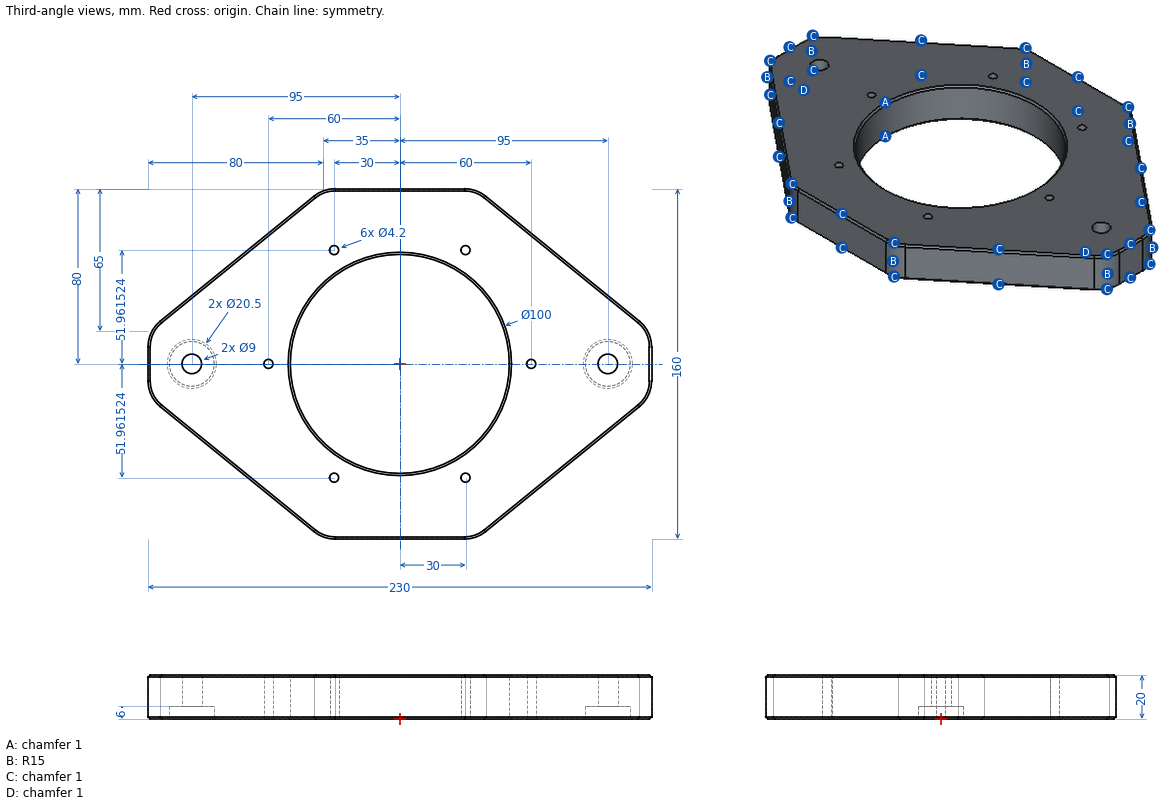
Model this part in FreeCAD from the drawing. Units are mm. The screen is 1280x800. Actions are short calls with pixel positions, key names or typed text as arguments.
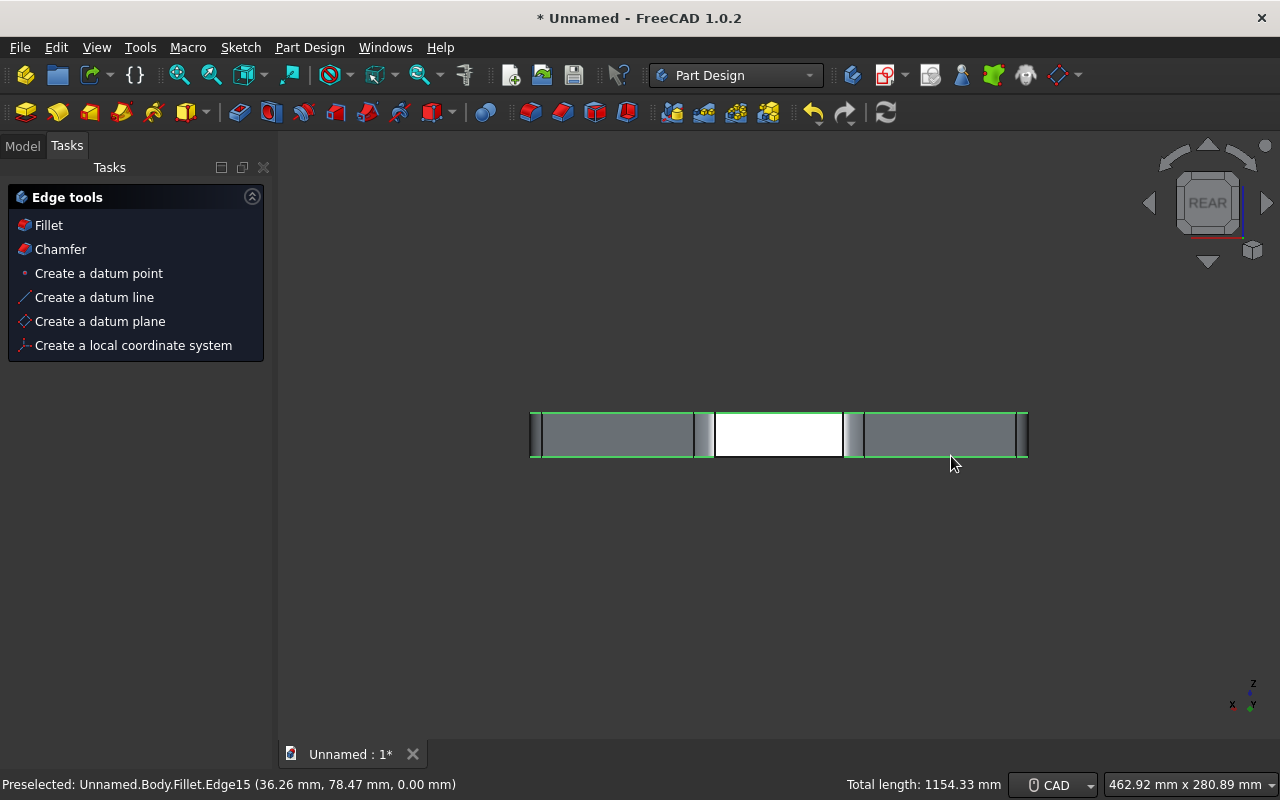
click(779, 456, ctrl)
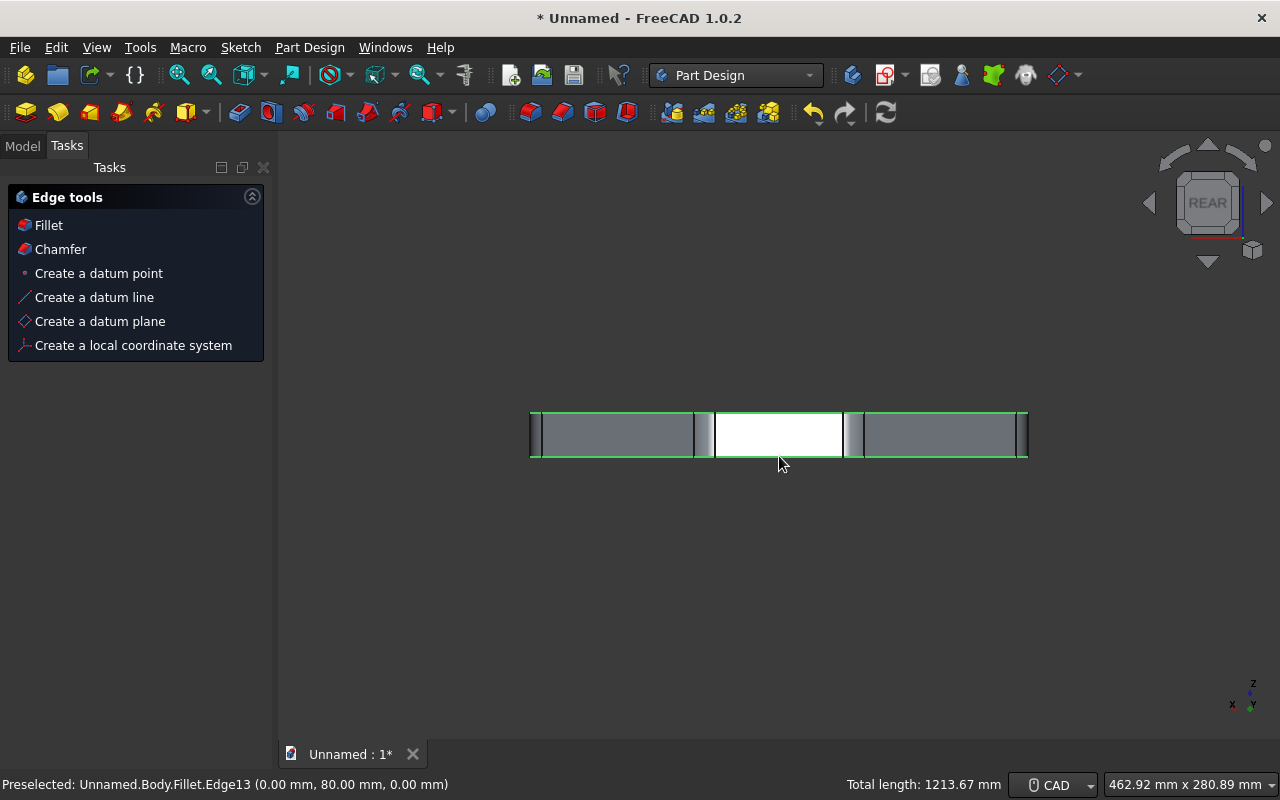
click(564, 112)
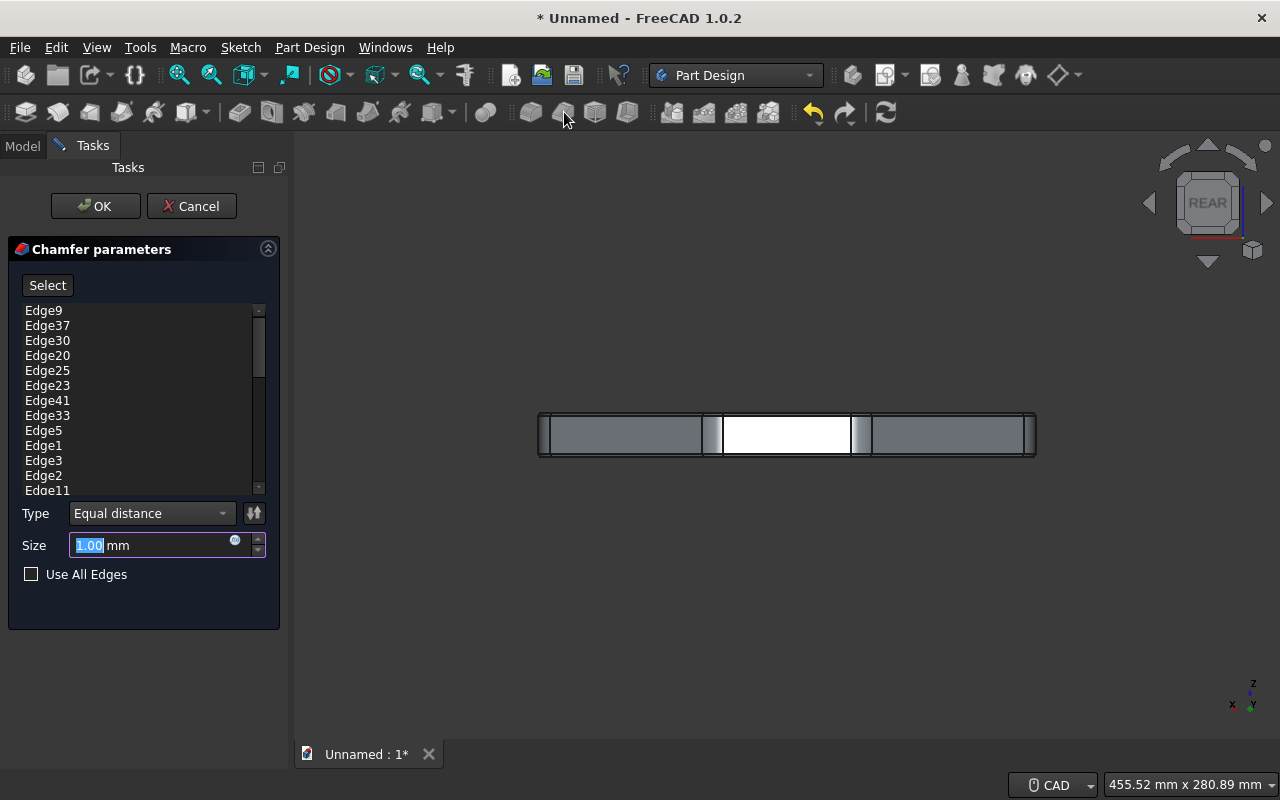
text(1)
key(Tab)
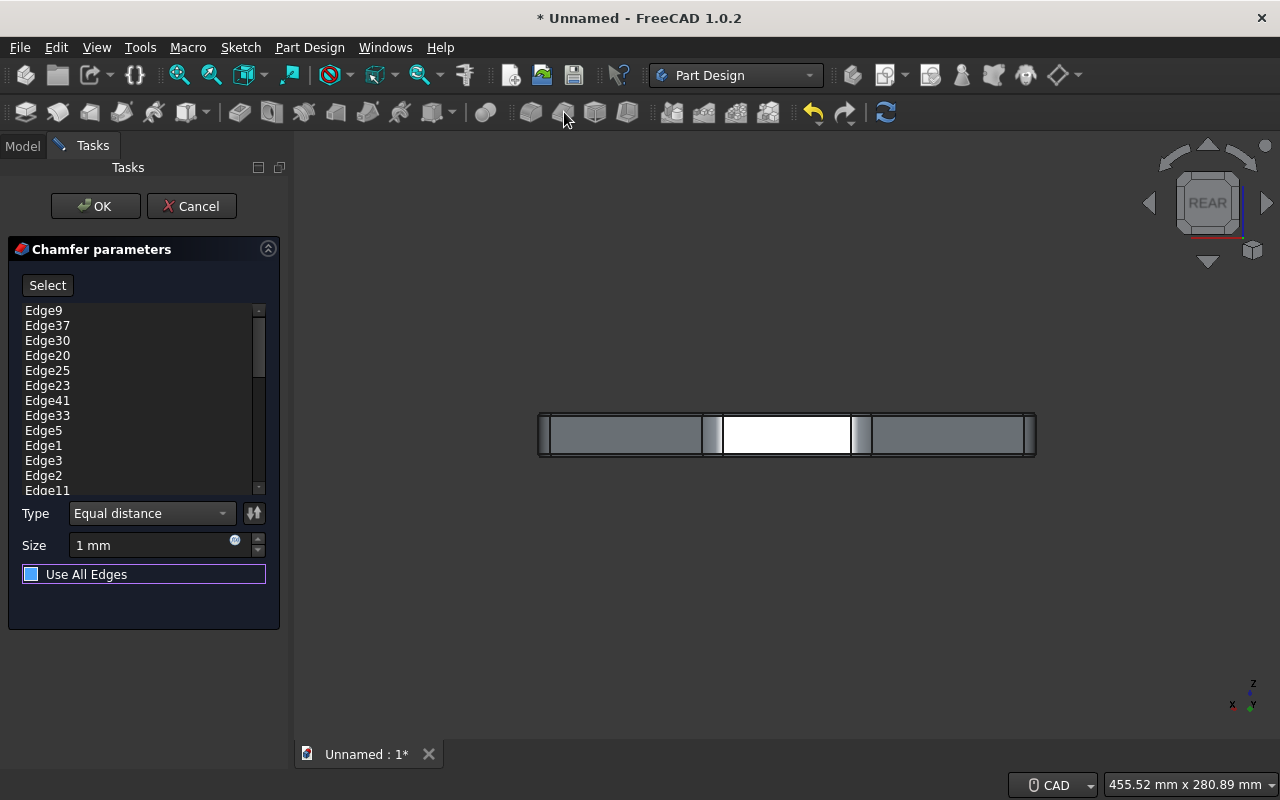
click(96, 206)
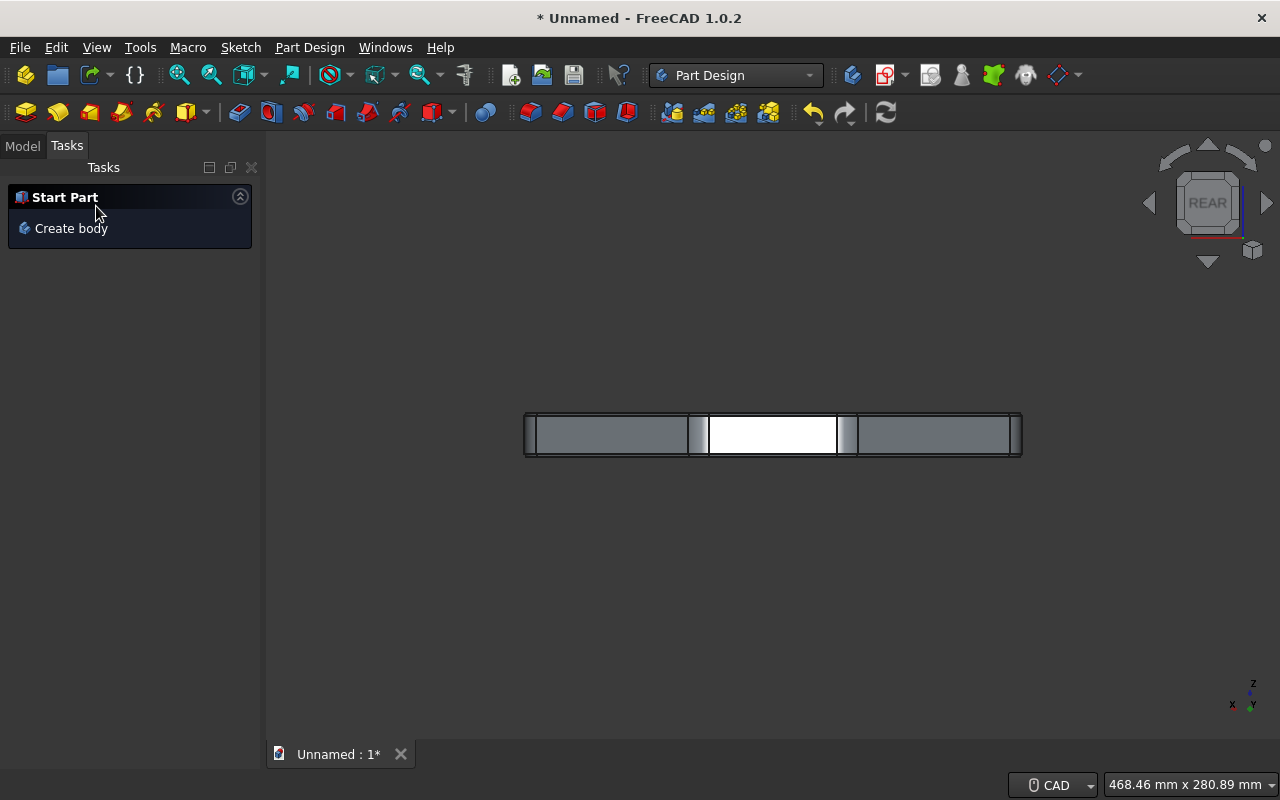
key(0)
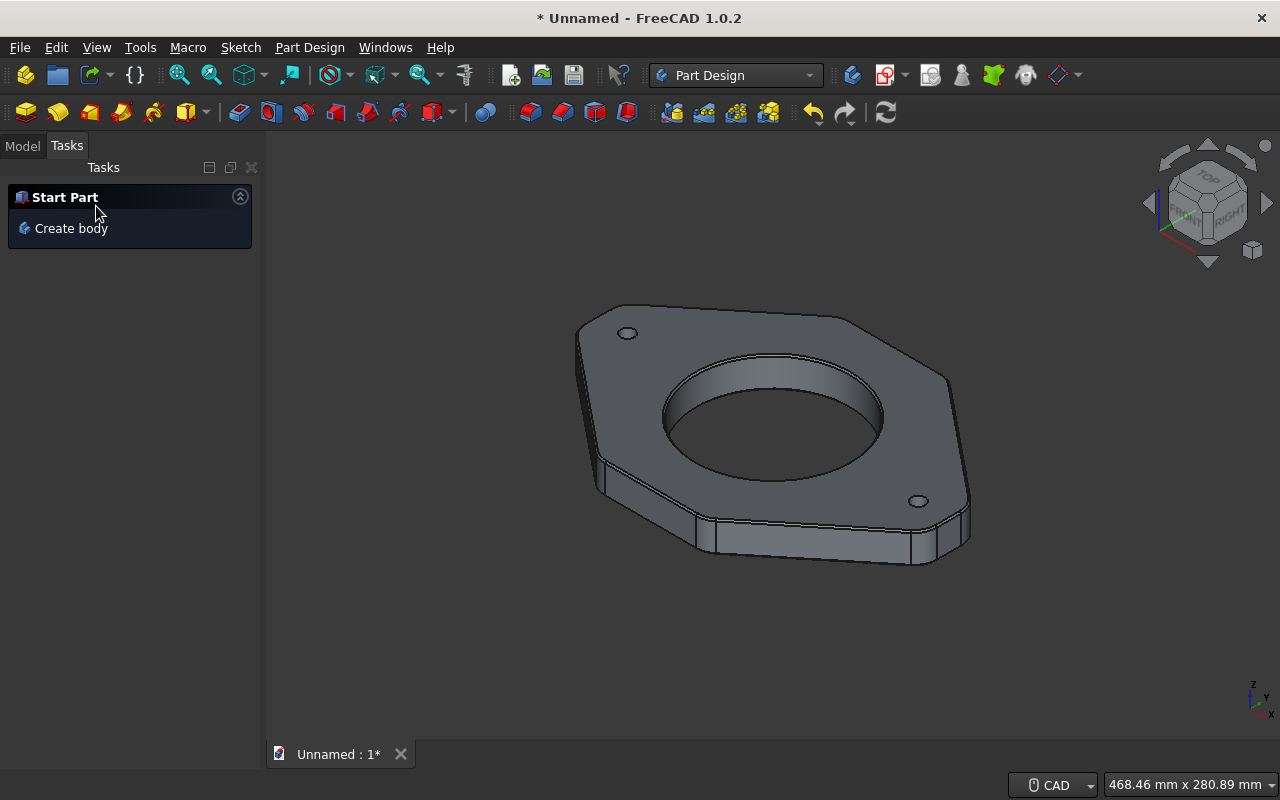
key(2)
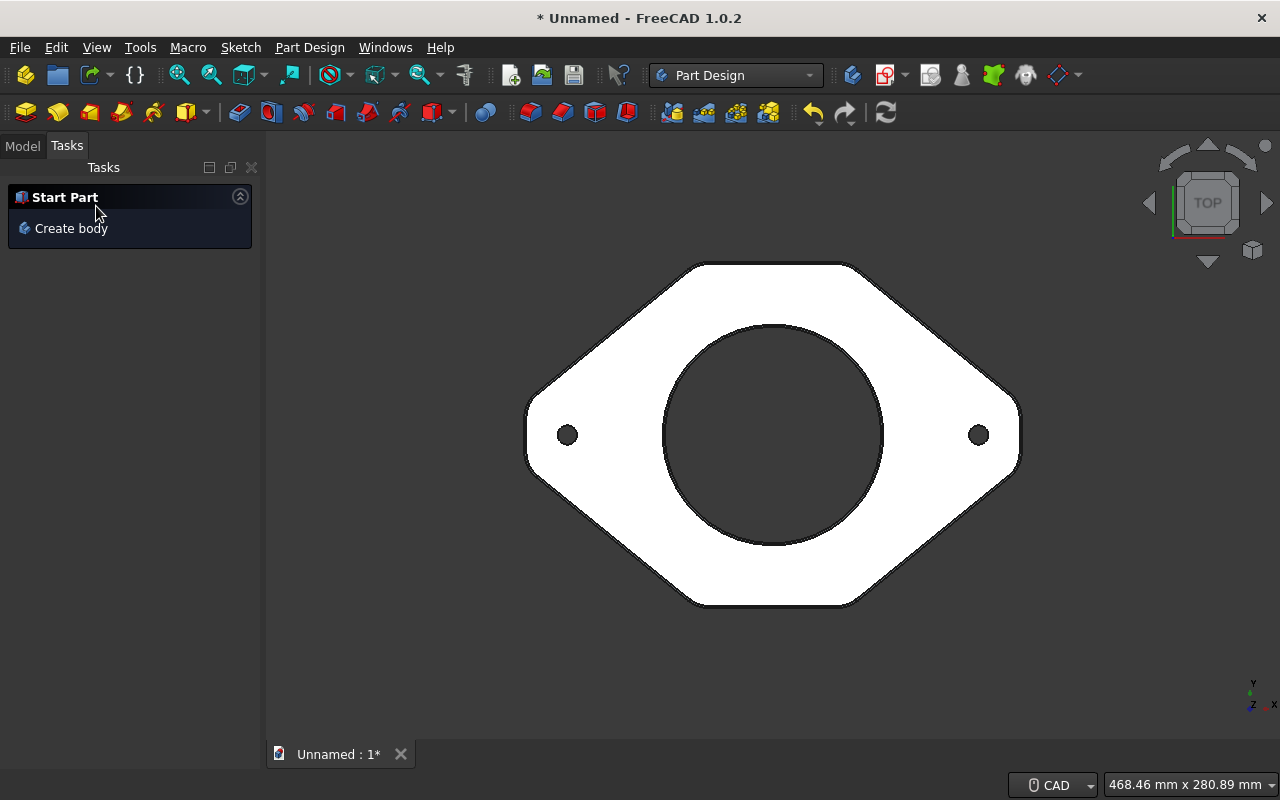
key(1)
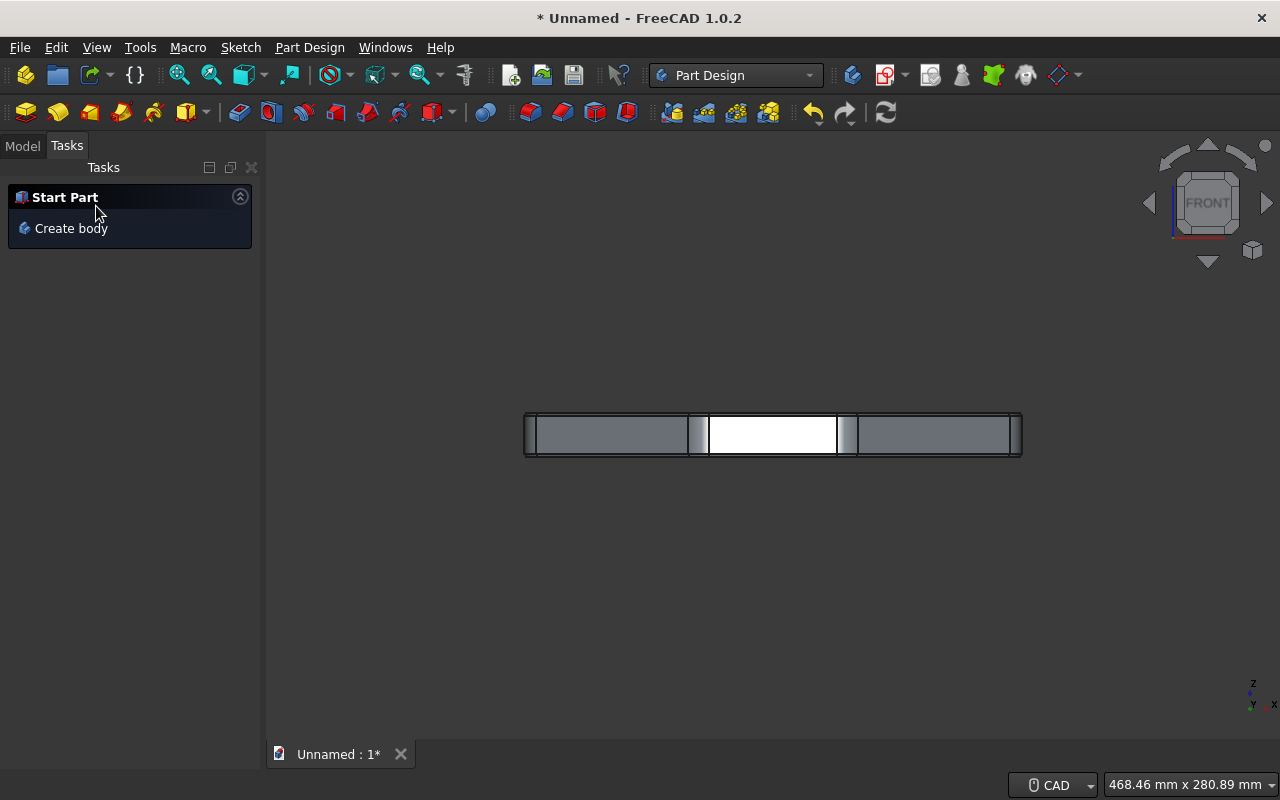
key(3)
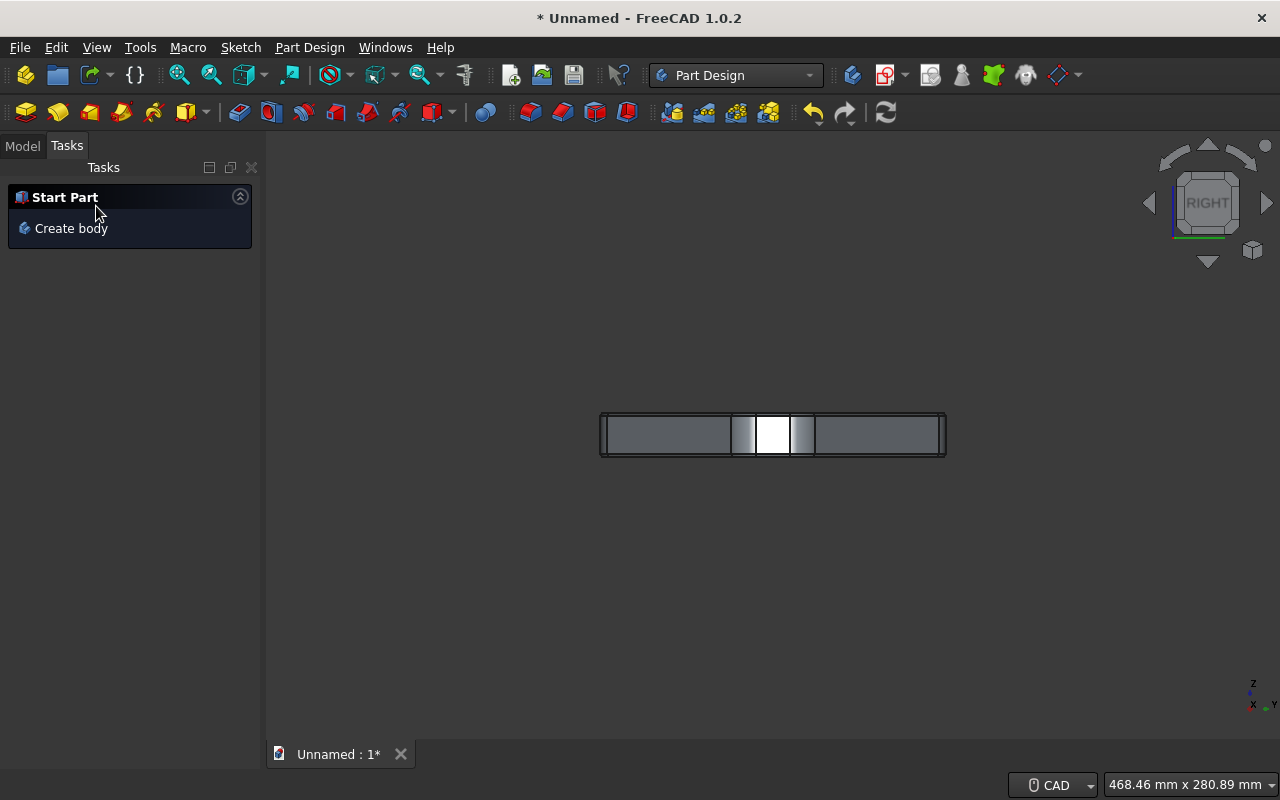
click(180, 76)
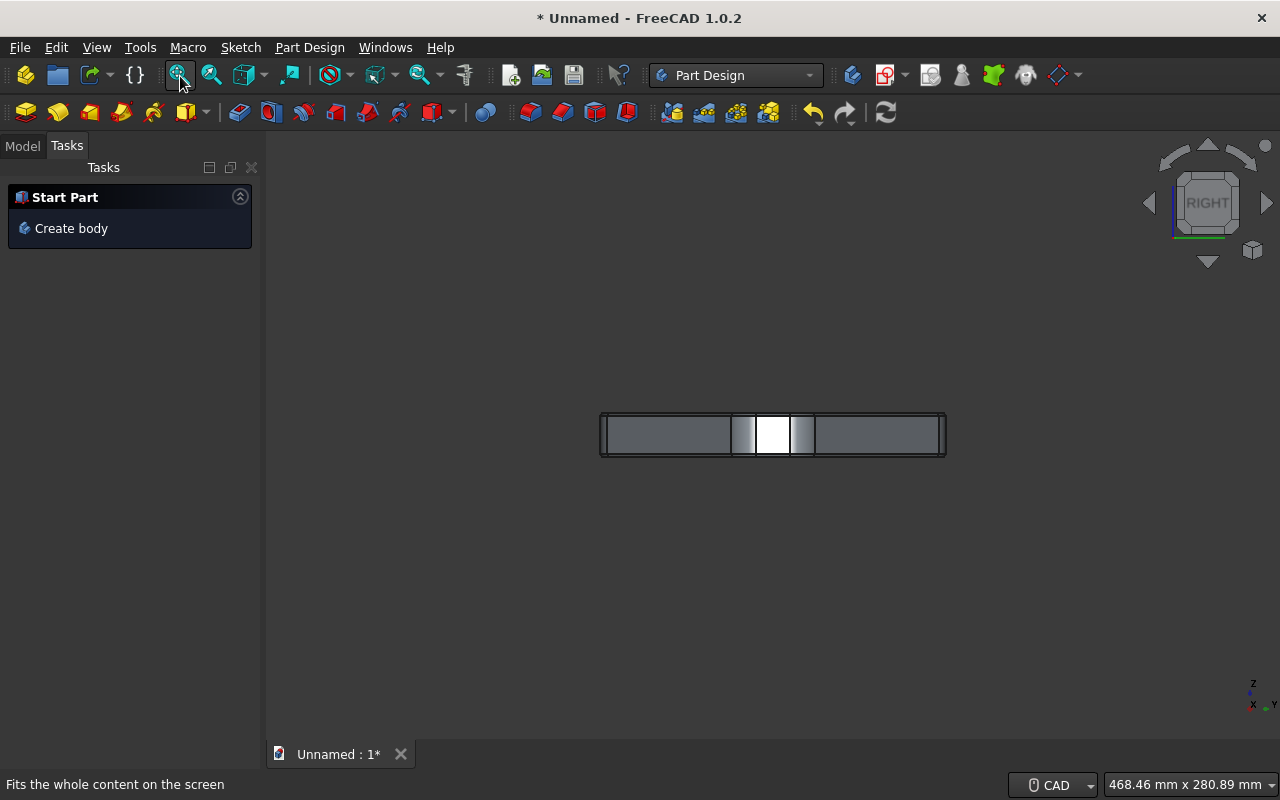
key(5)